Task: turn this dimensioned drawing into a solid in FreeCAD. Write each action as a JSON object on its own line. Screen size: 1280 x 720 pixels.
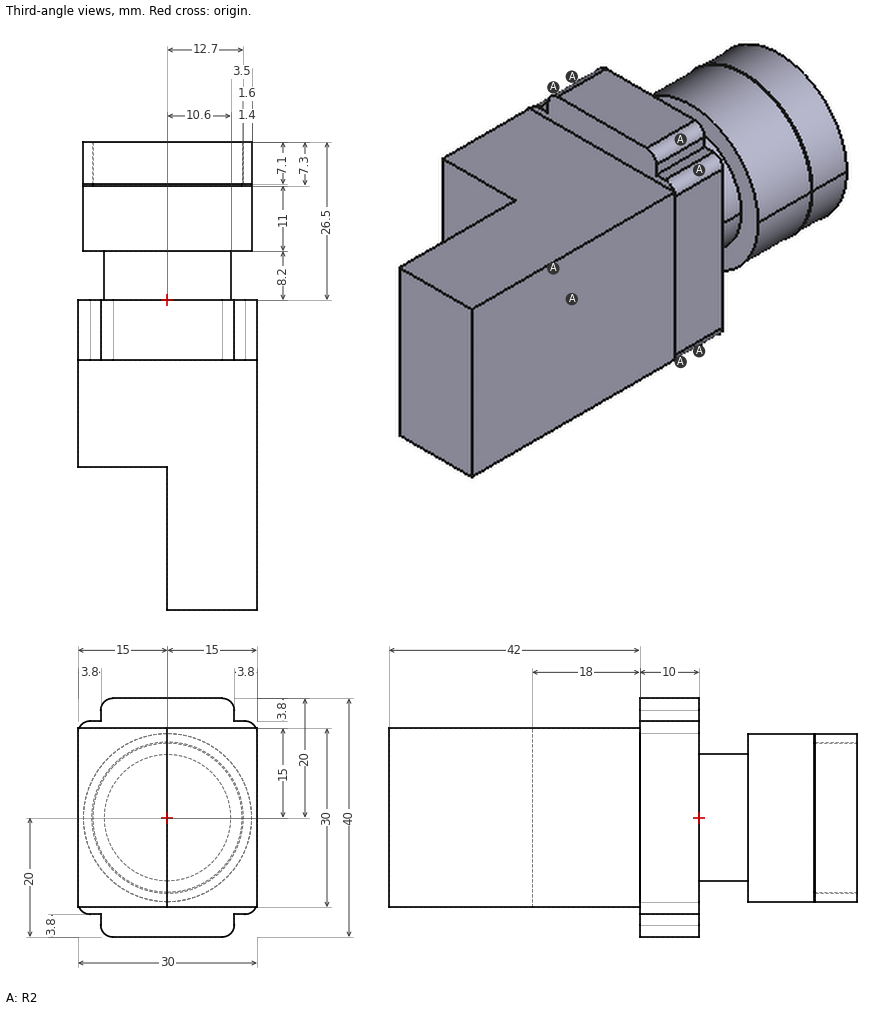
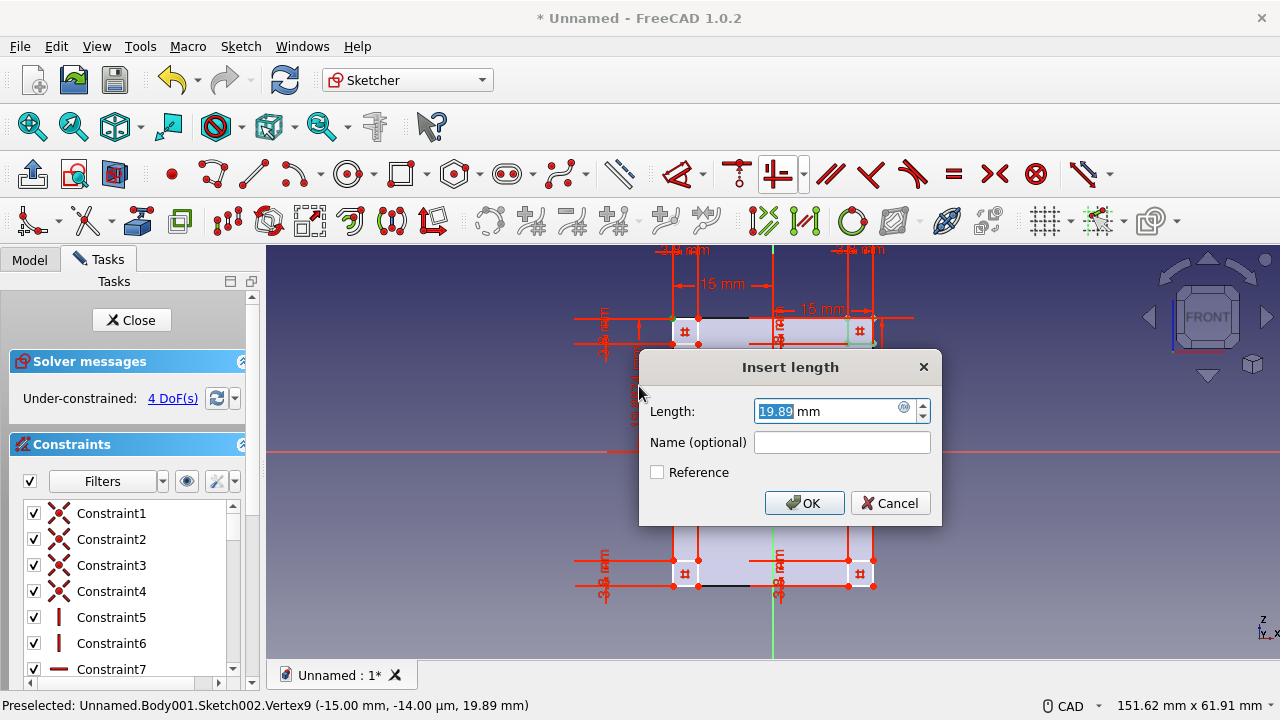
{"action": "type", "text": "20"}
{"action": "key", "text": "Return"}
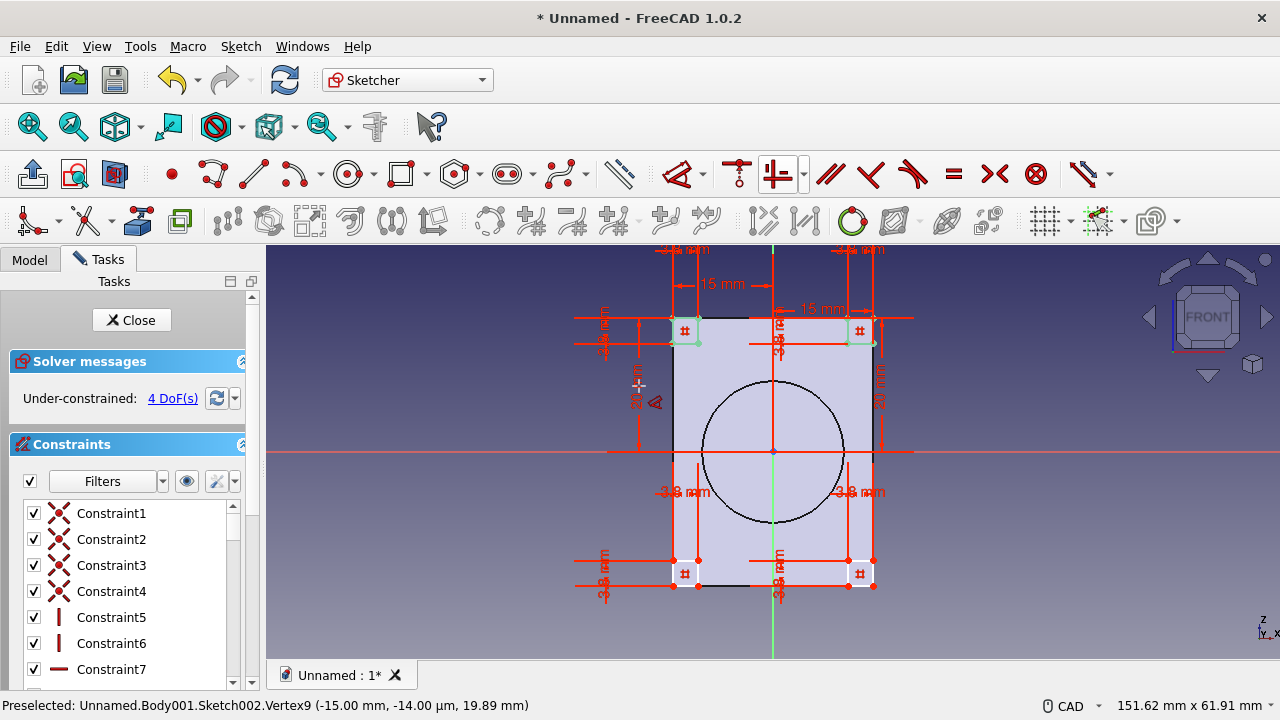
{"action": "left_click", "coordinate": [673, 561]}
{"action": "left_click", "coordinate": [723, 595]}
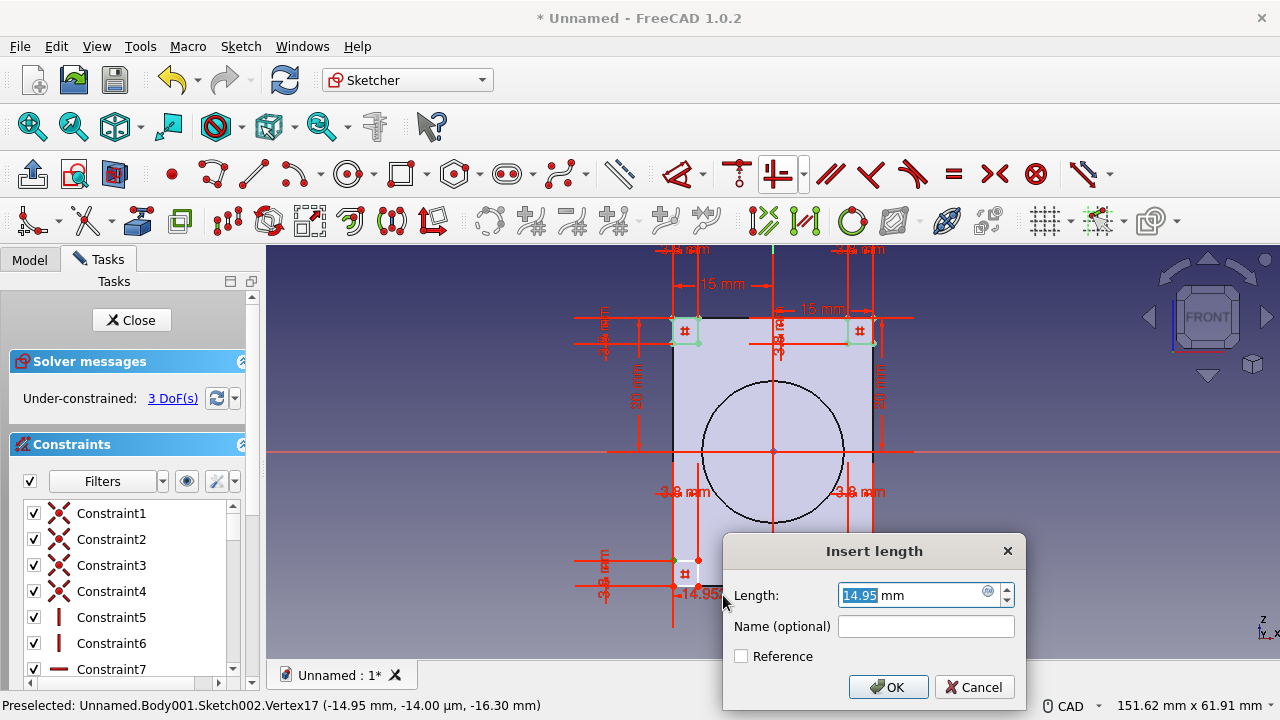
{"action": "type", "text": "15"}
{"action": "key", "text": "Return"}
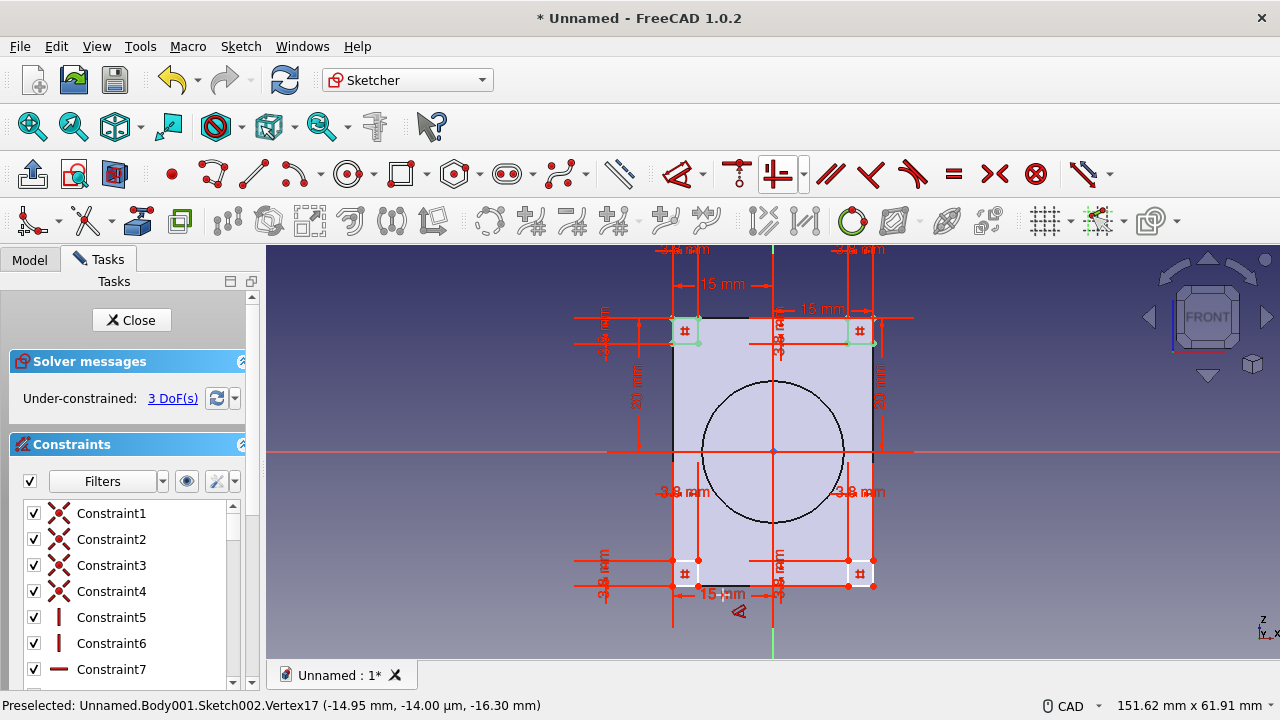
{"action": "left_click", "coordinate": [673, 586]}
{"action": "left_click", "coordinate": [639, 519]}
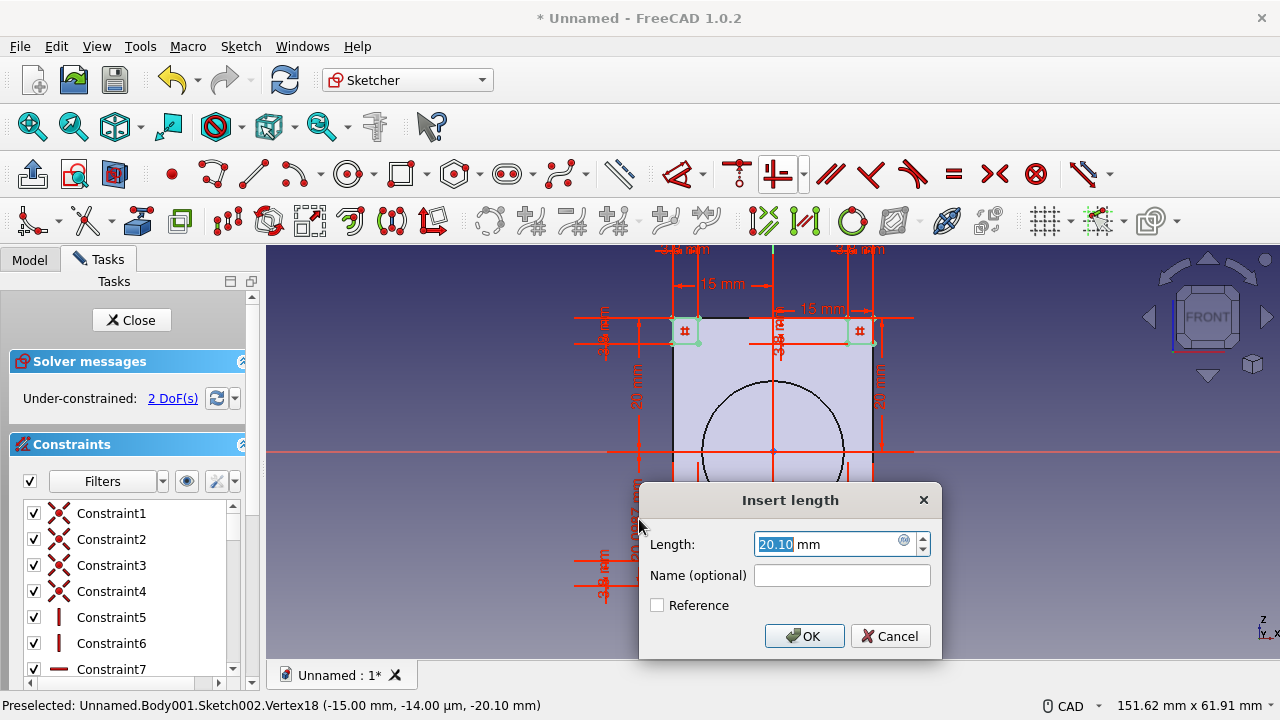
{"action": "type", "text": "20"}
{"action": "key", "text": "Return"}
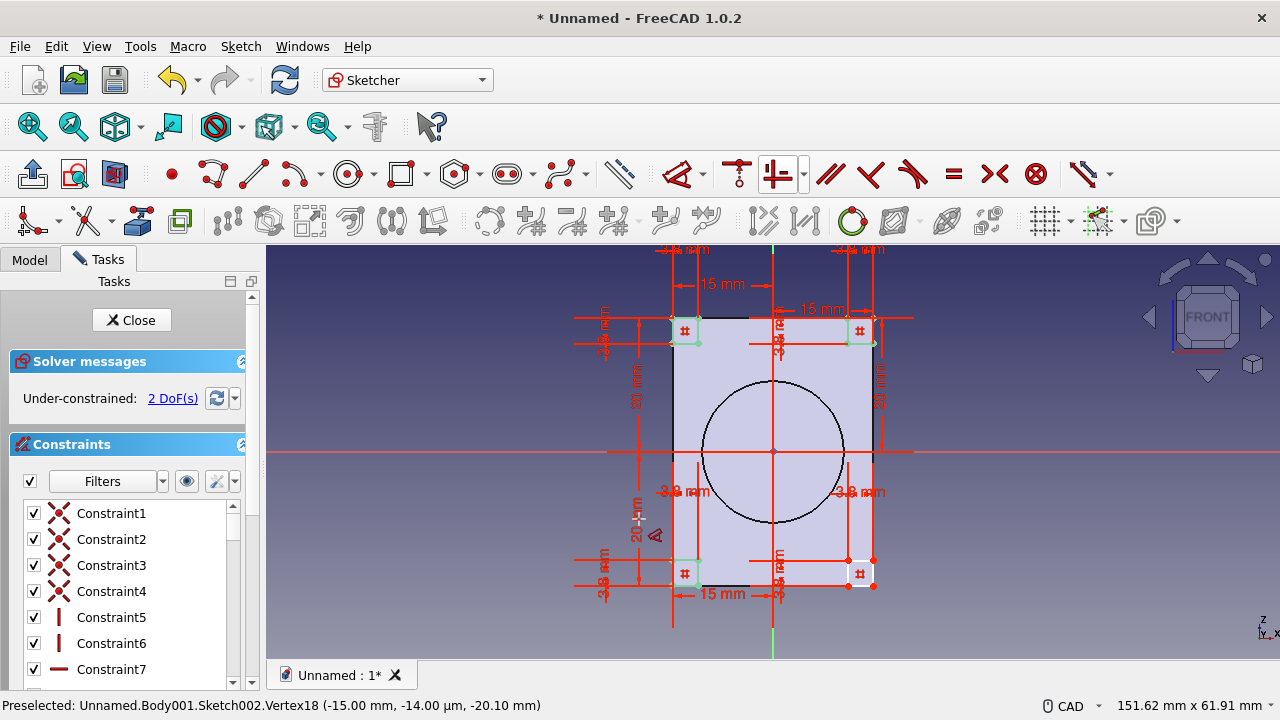
{"action": "left_click", "coordinate": [848, 586]}
{"action": "left_click", "coordinate": [882, 519]}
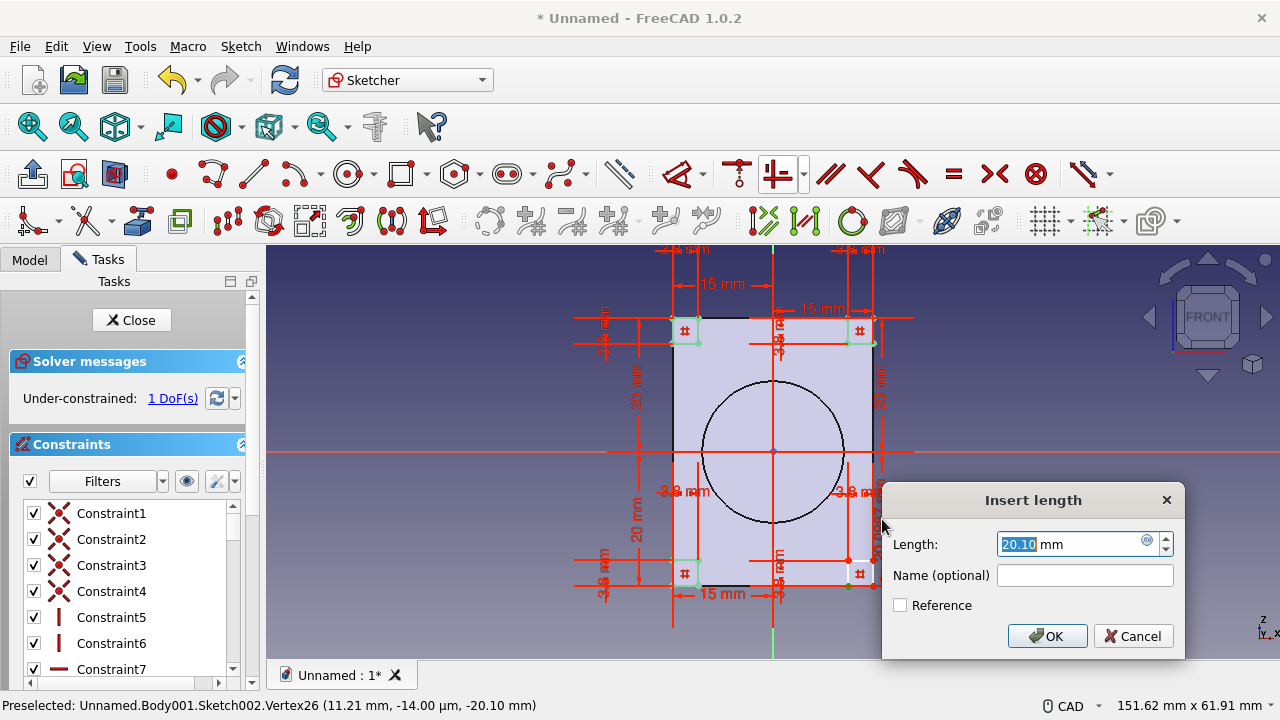
{"action": "type", "text": "20"}
{"action": "key", "text": "Return"}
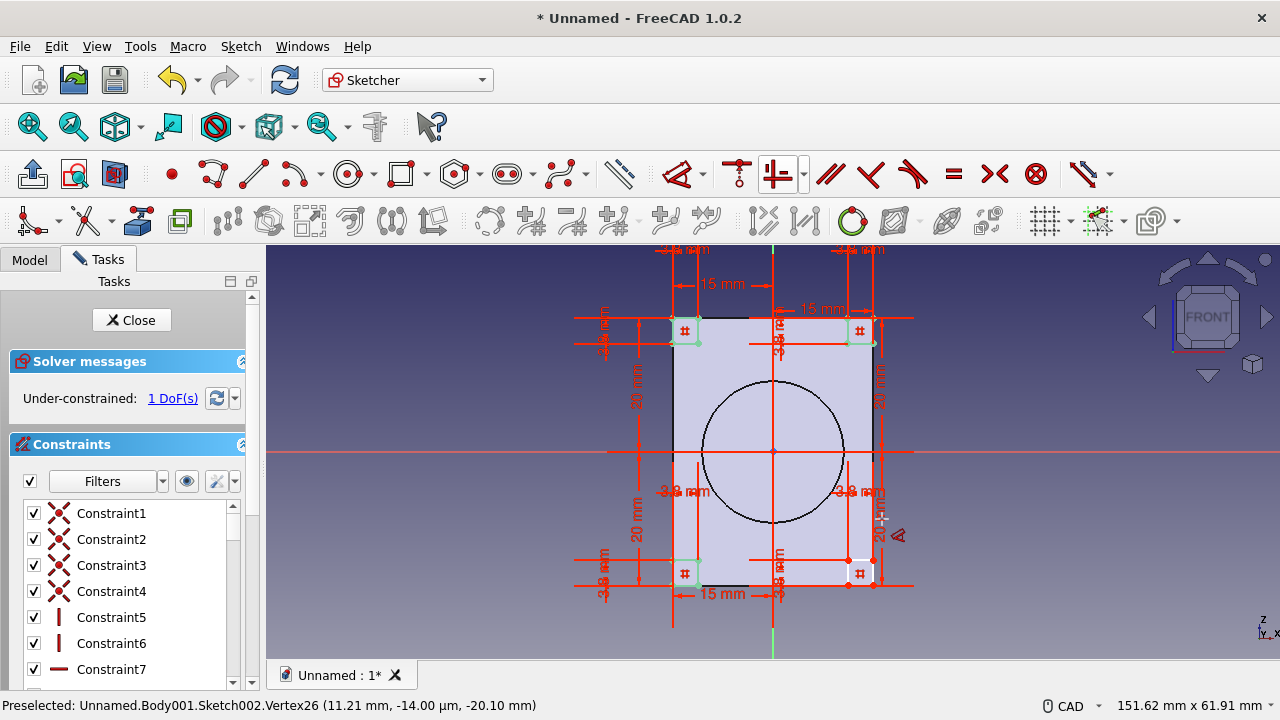
{"action": "left_click", "coordinate": [873, 586]}
{"action": "left_click", "coordinate": [823, 620]}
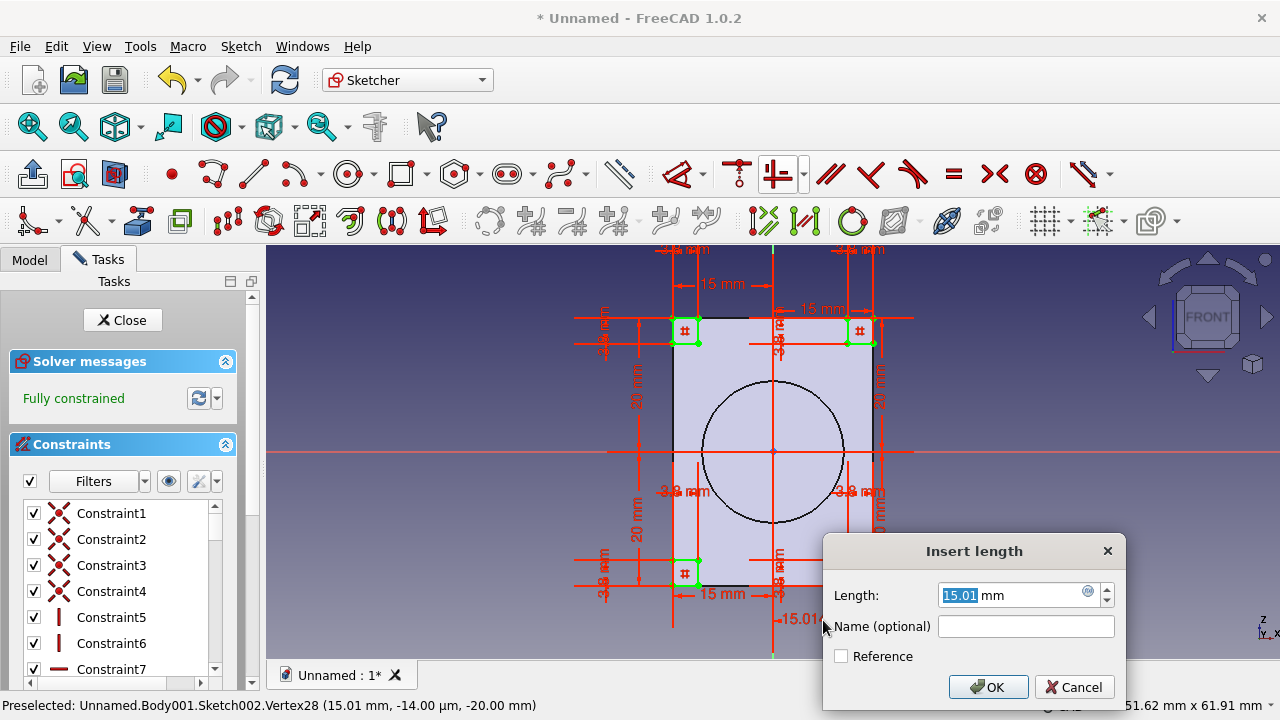
{"action": "type", "text": "15"}
{"action": "key", "text": "Return"}
{"action": "key", "text": "Escape"}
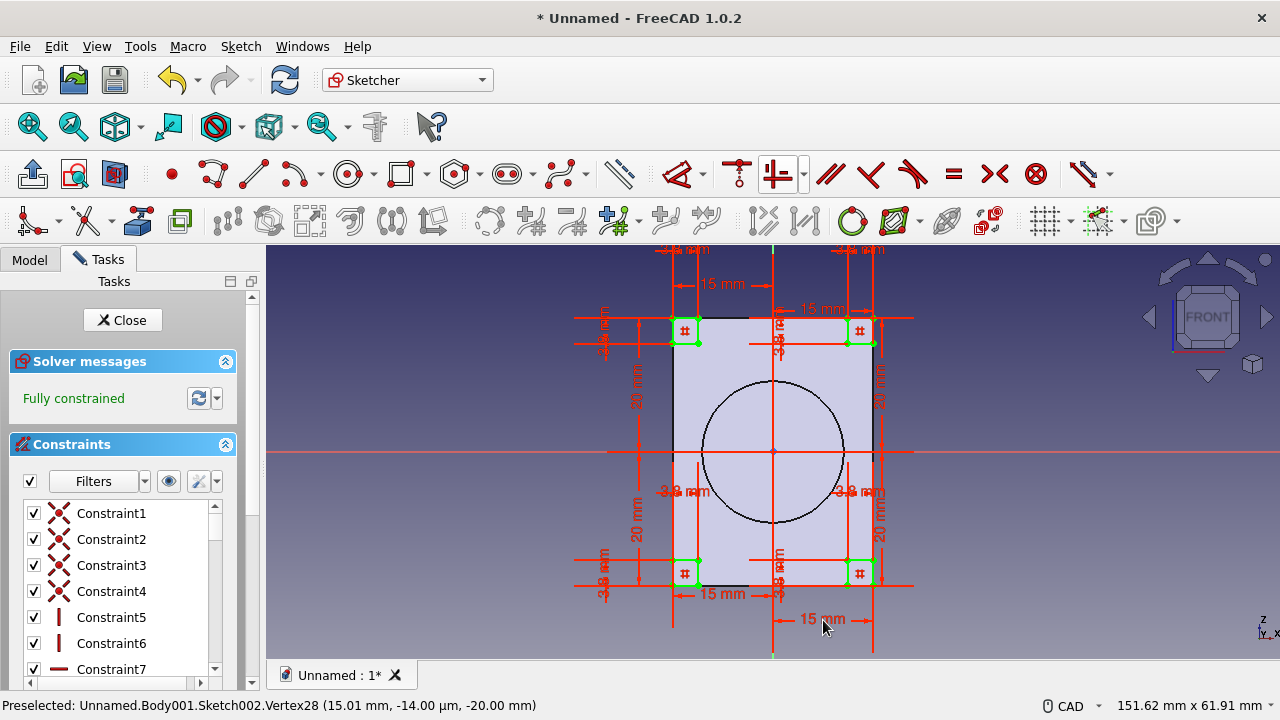
{"action": "left_click", "coordinate": [123, 320]}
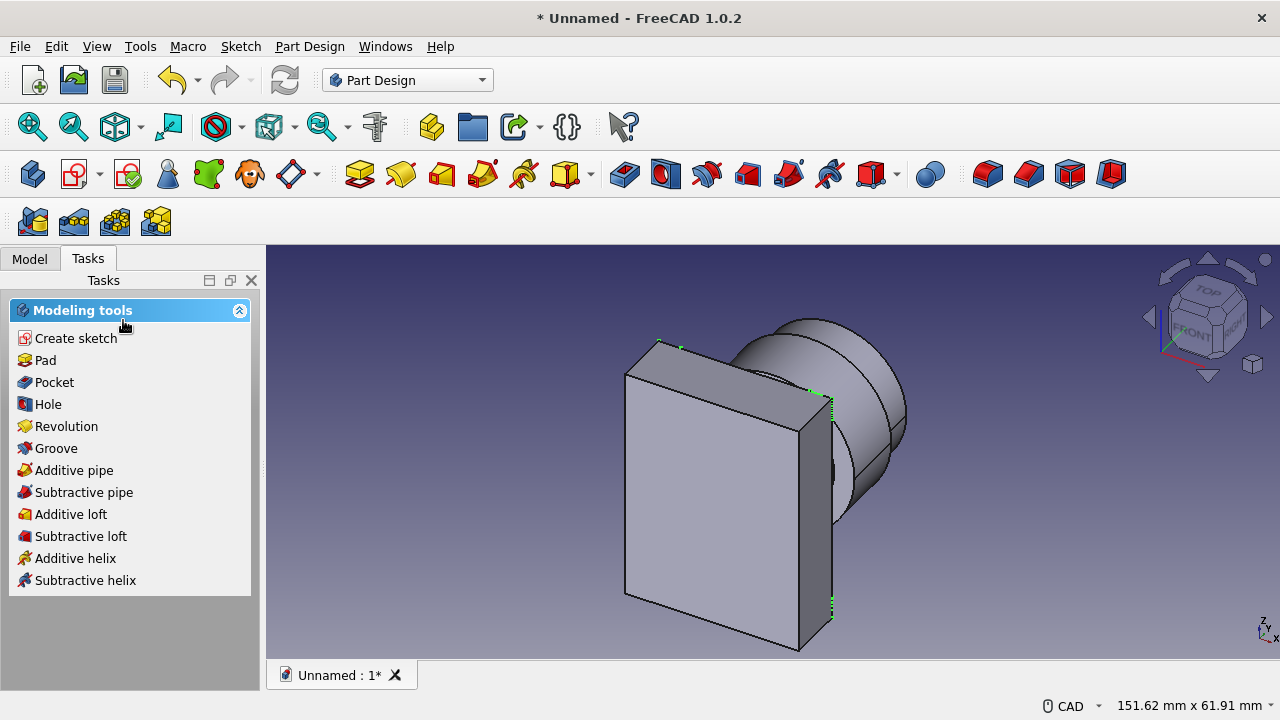
{"action": "left_click", "coordinate": [625, 174]}